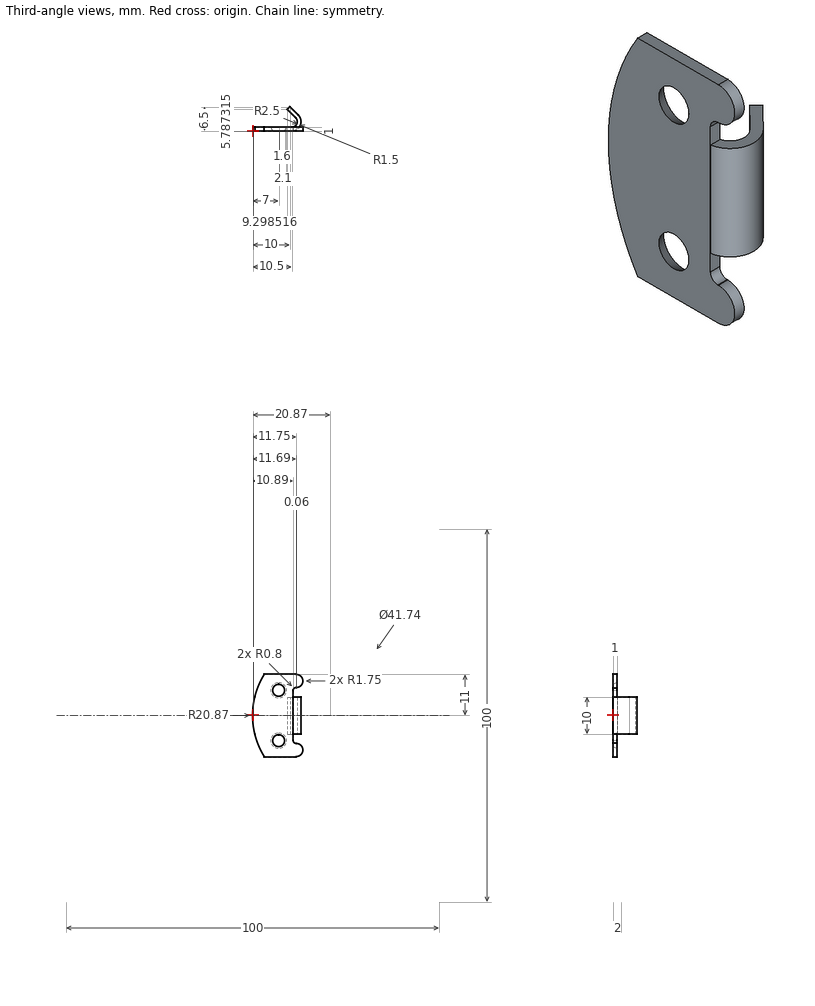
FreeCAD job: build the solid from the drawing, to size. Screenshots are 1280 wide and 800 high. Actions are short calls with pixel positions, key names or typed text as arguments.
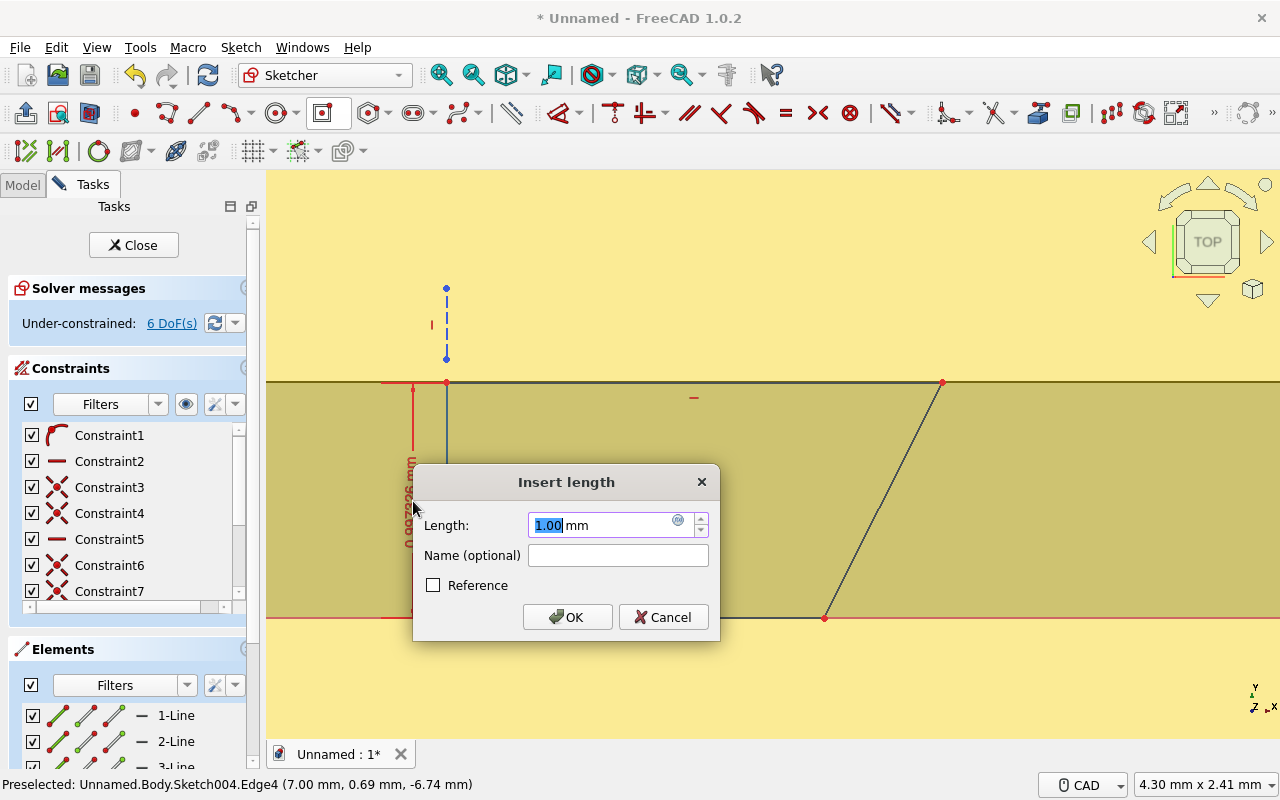
text(1)
key(Return)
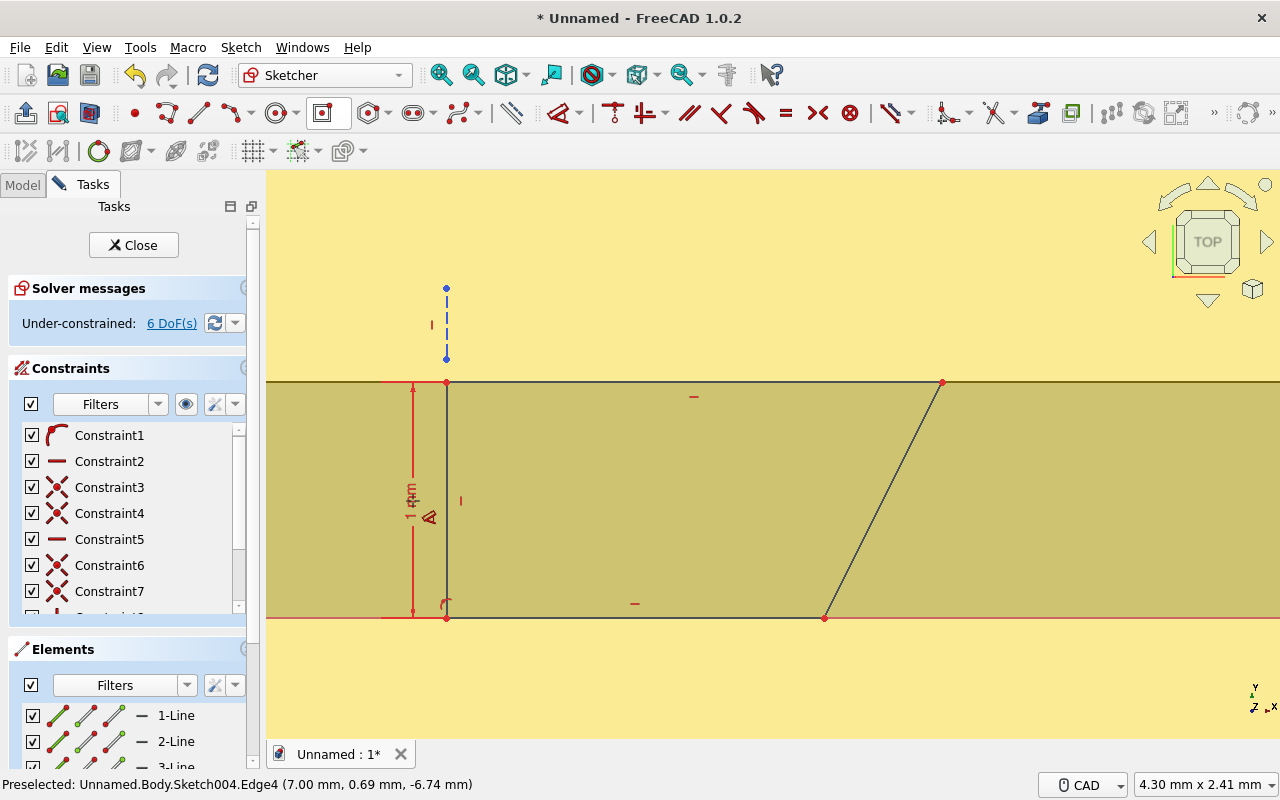
click(447, 618)
click(370, 652)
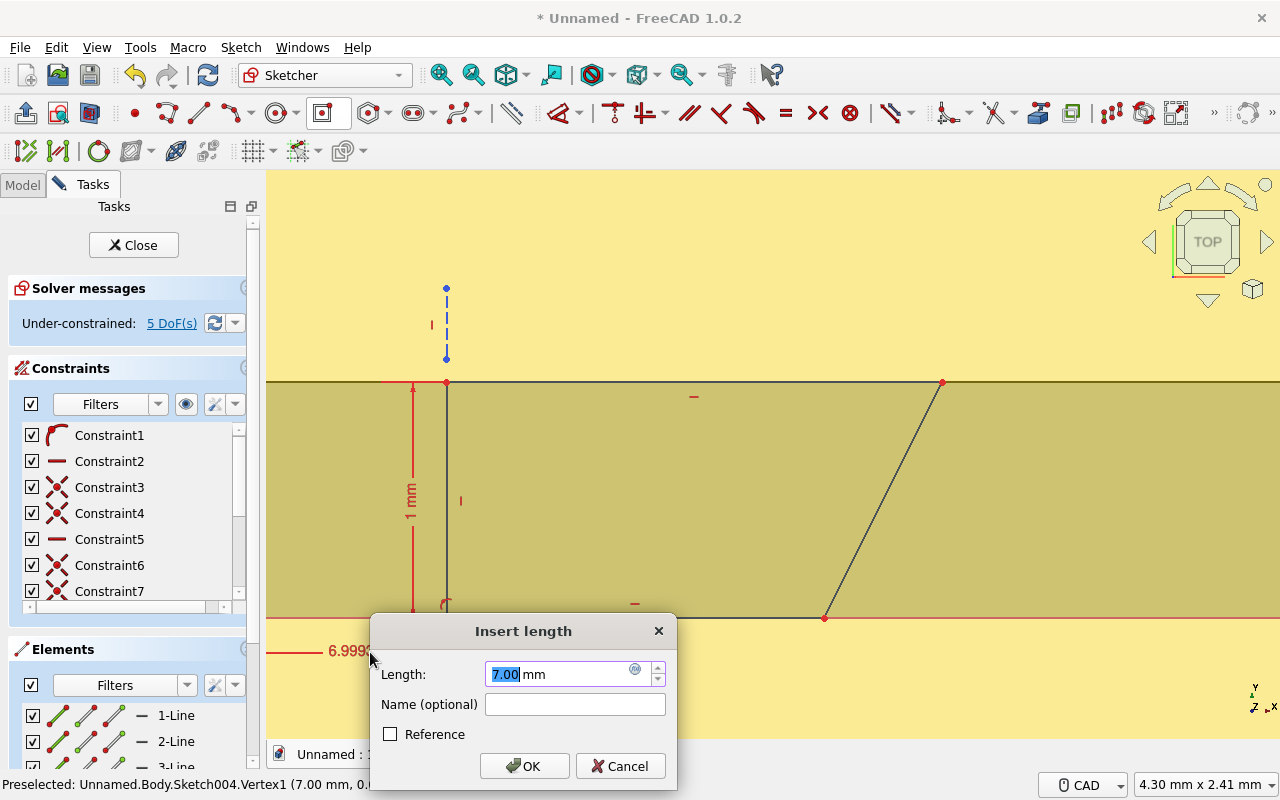
text(7)
key(Return)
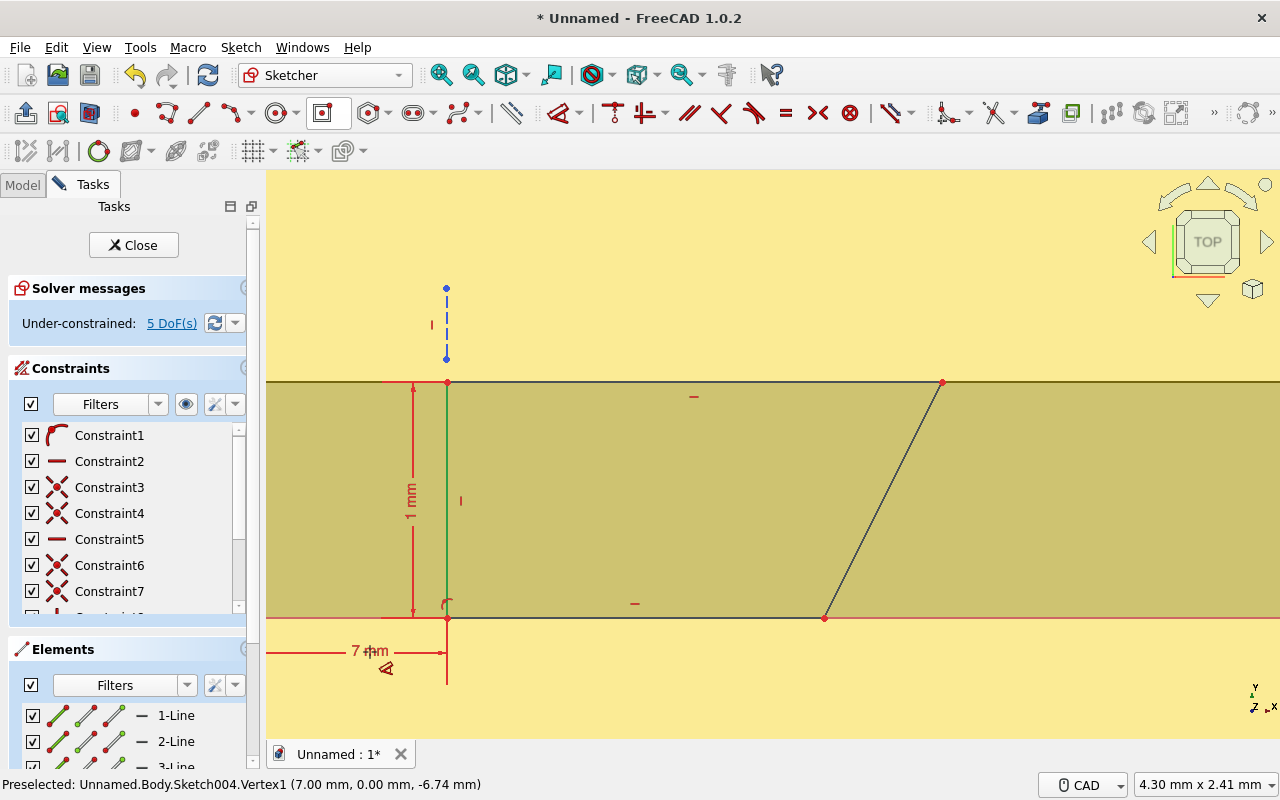
click(447, 360)
click(370, 326)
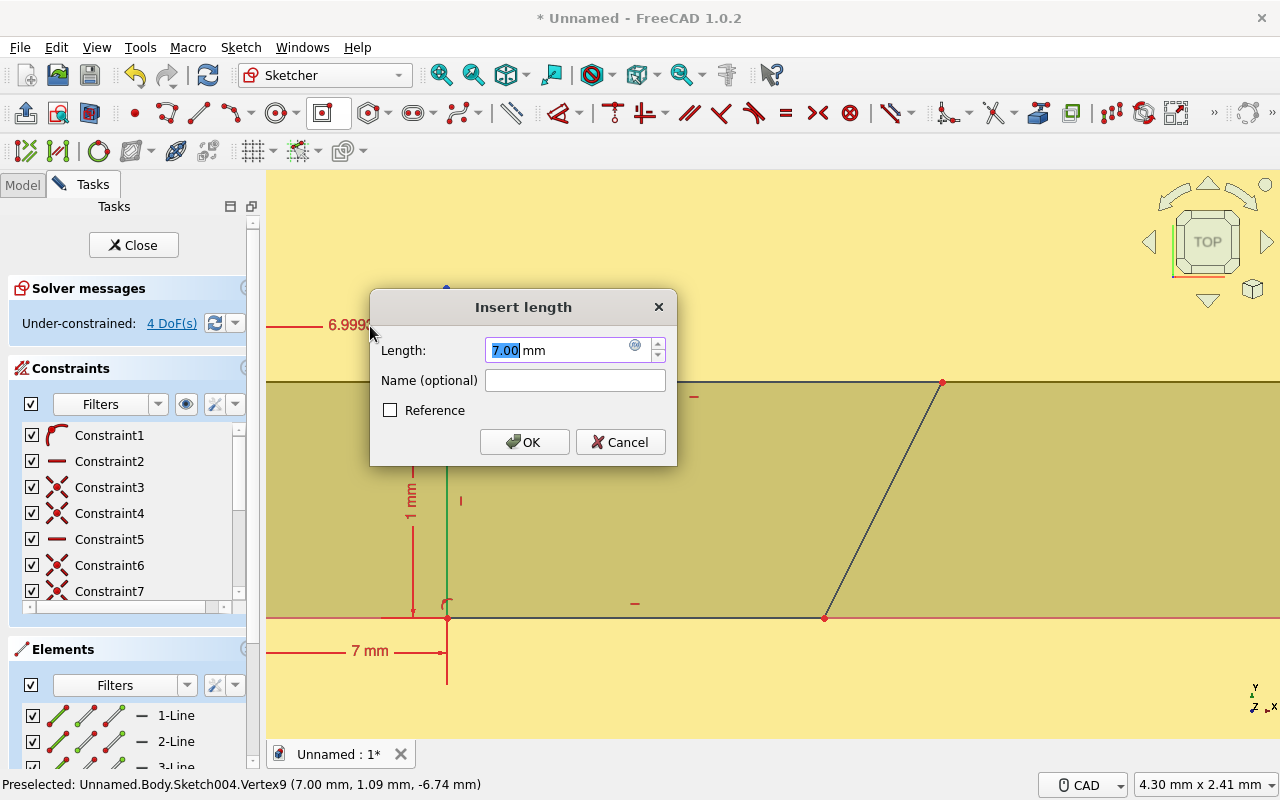
text(7)
key(Return)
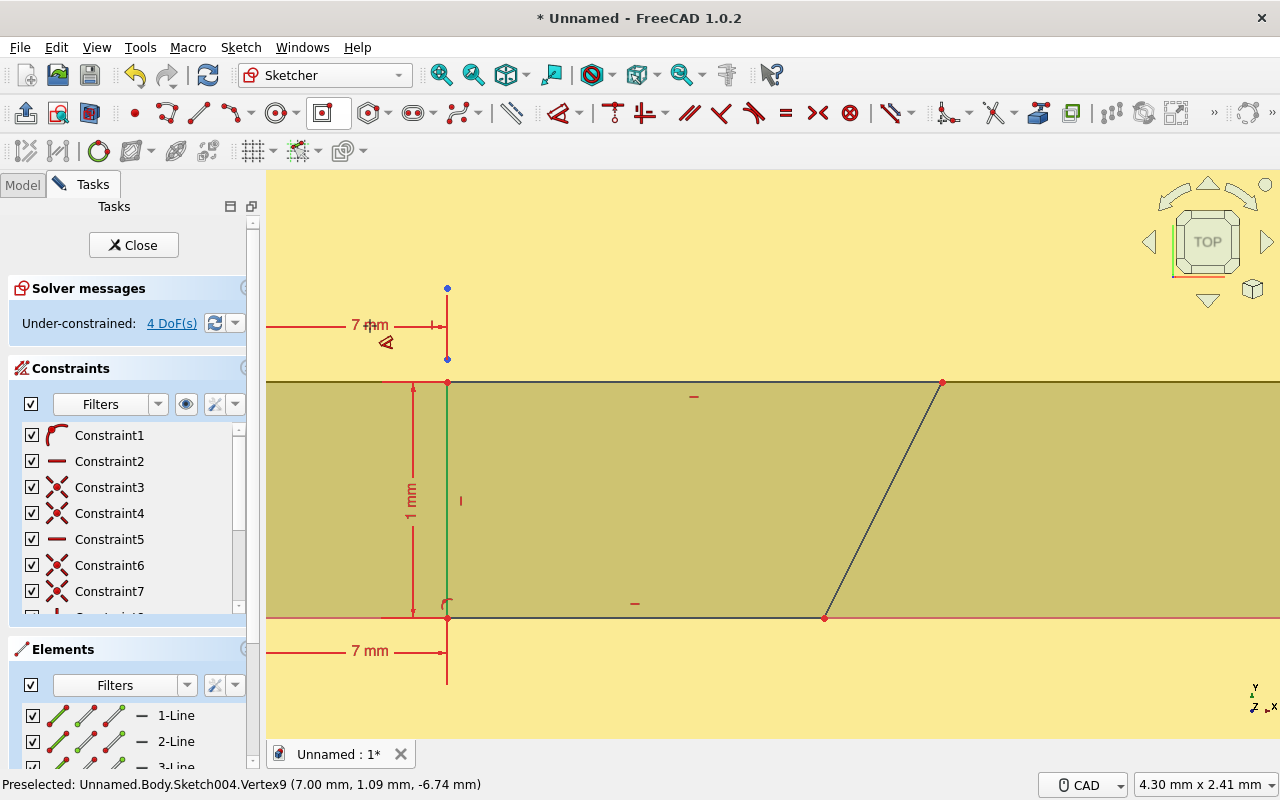
click(560, 618)
click(636, 652)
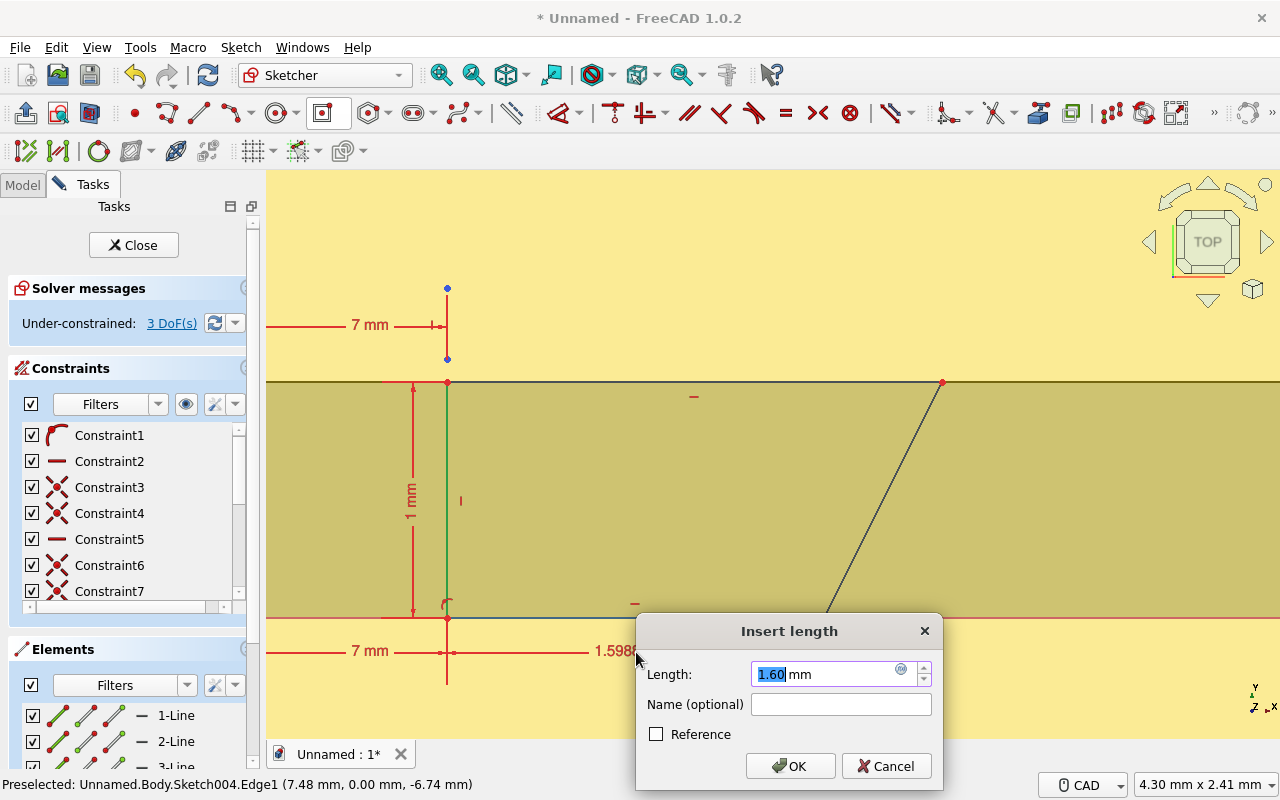
text(1.6)
key(Return)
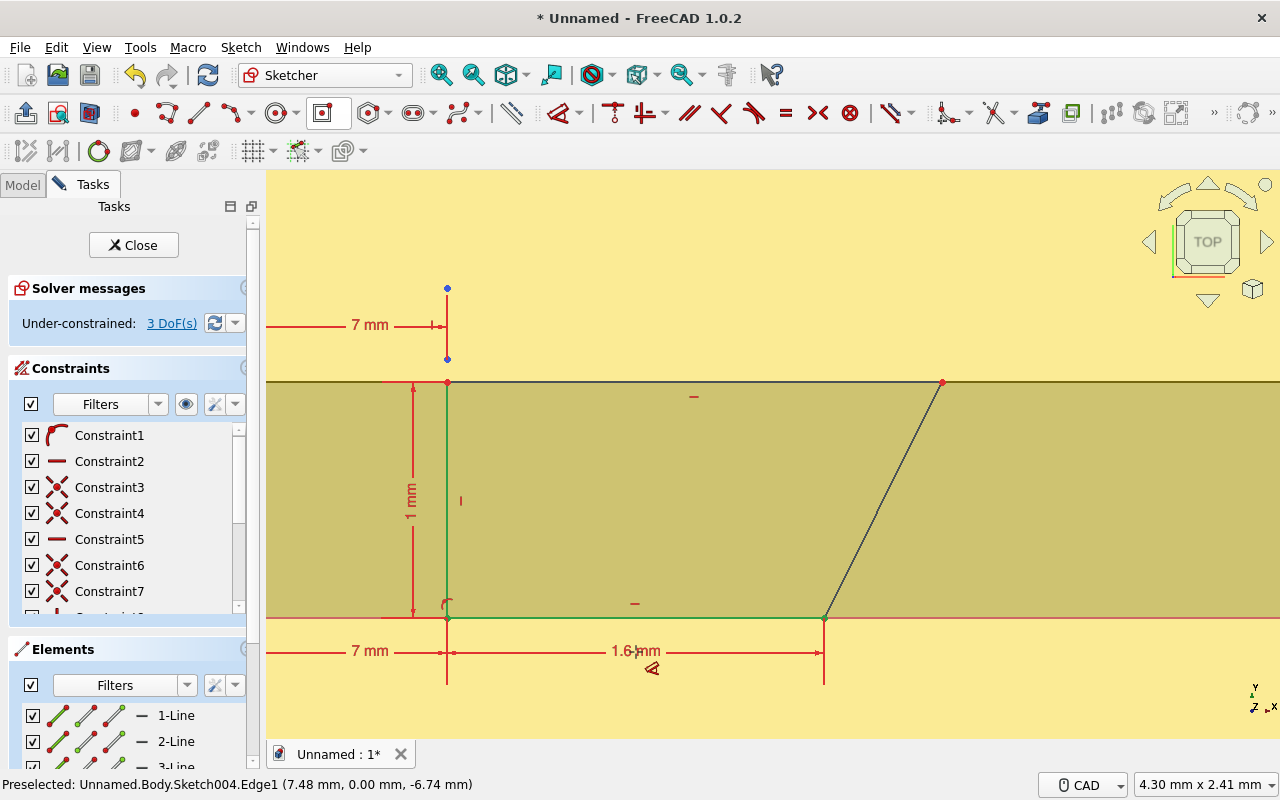
click(794, 382)
click(695, 348)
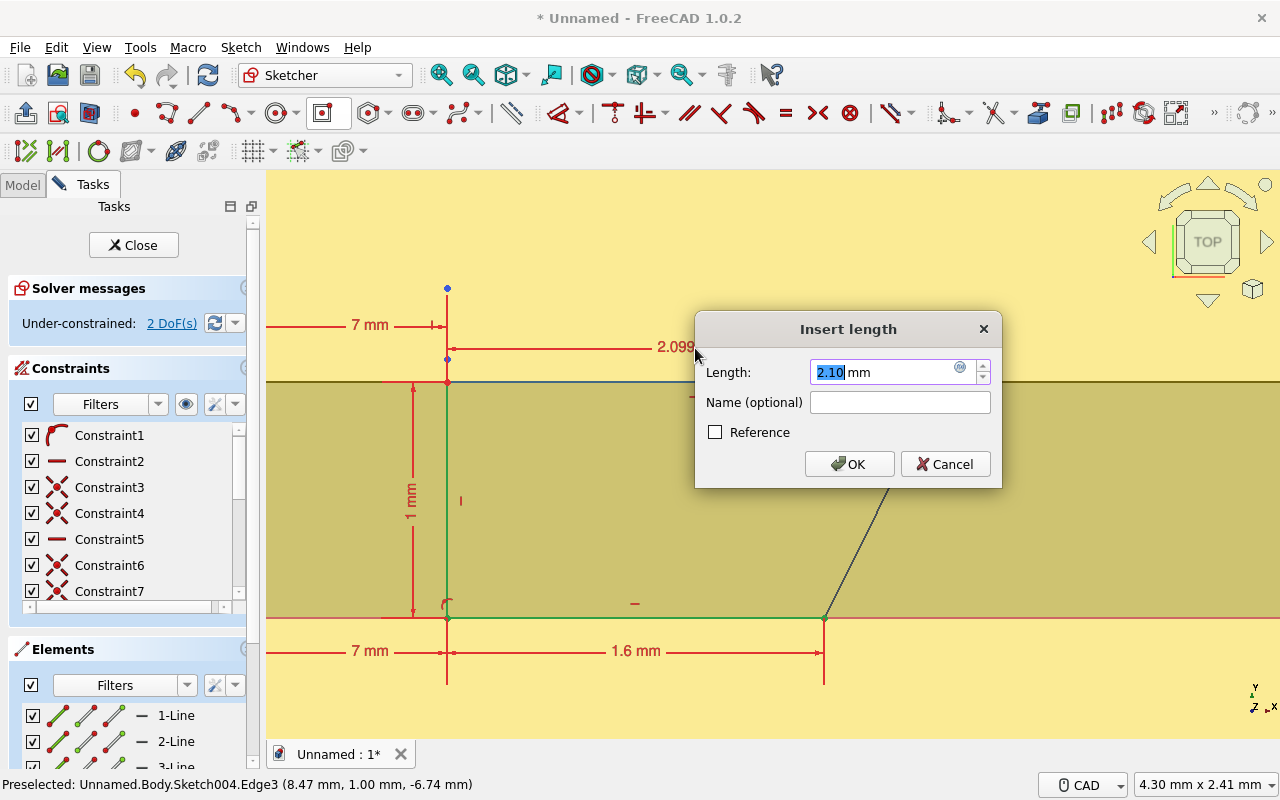
text(2.1)
key(Return)
key(Escape)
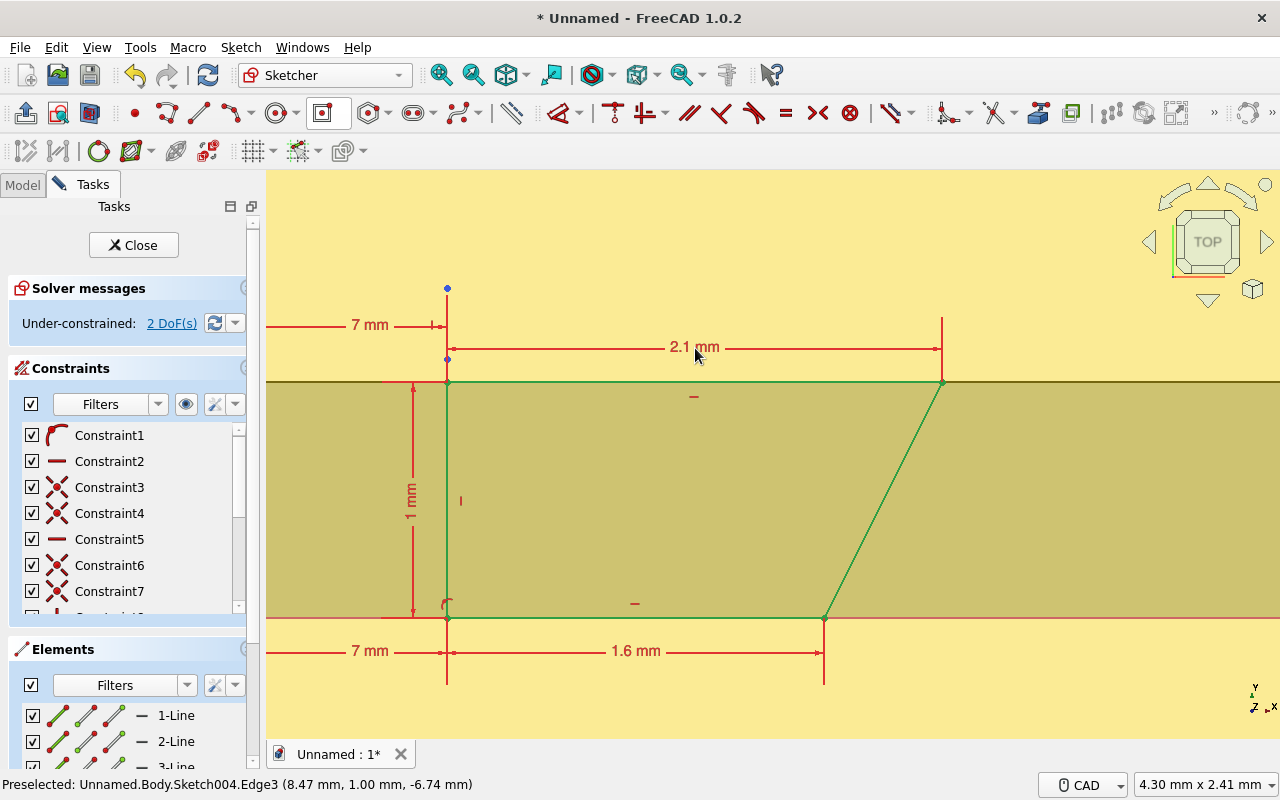
click(134, 245)